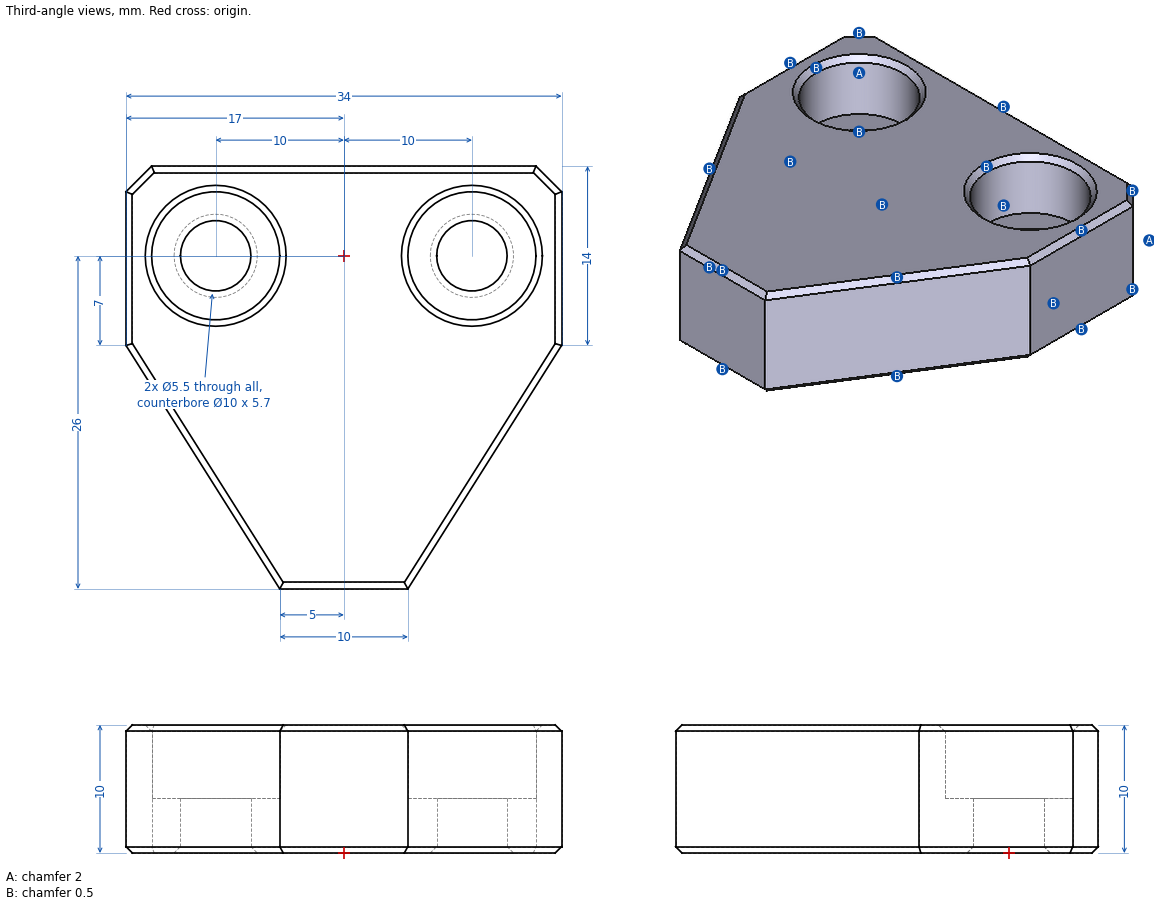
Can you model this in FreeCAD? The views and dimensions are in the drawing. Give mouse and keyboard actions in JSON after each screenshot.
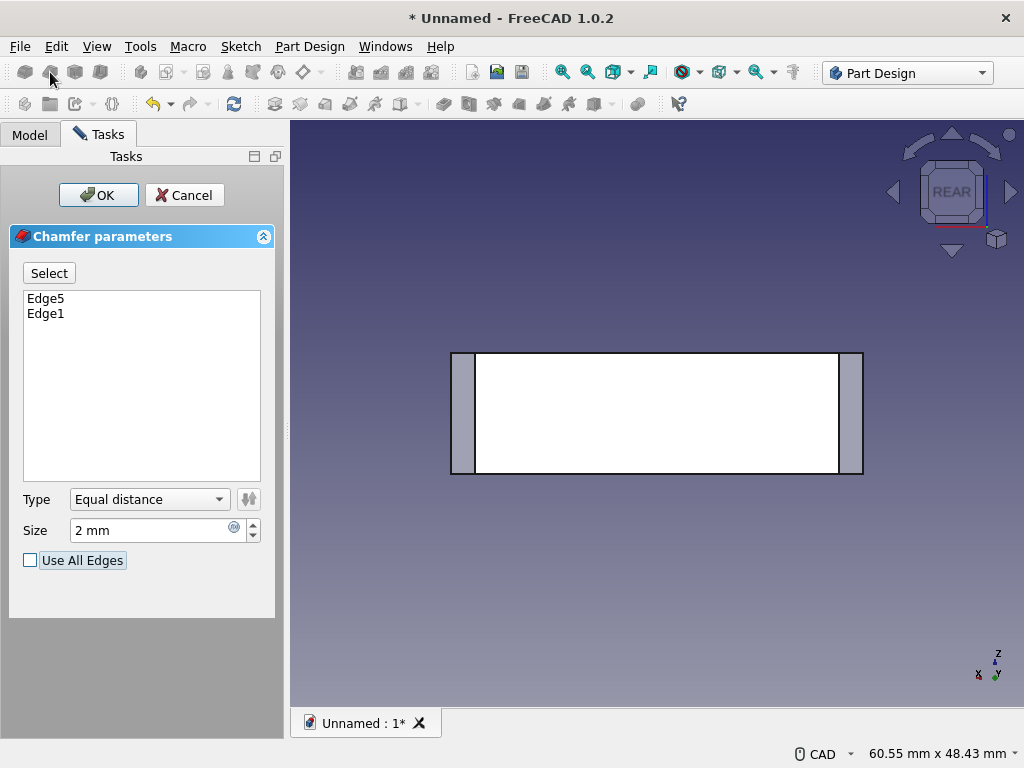
{"action": "left_click", "coordinate": [99, 195]}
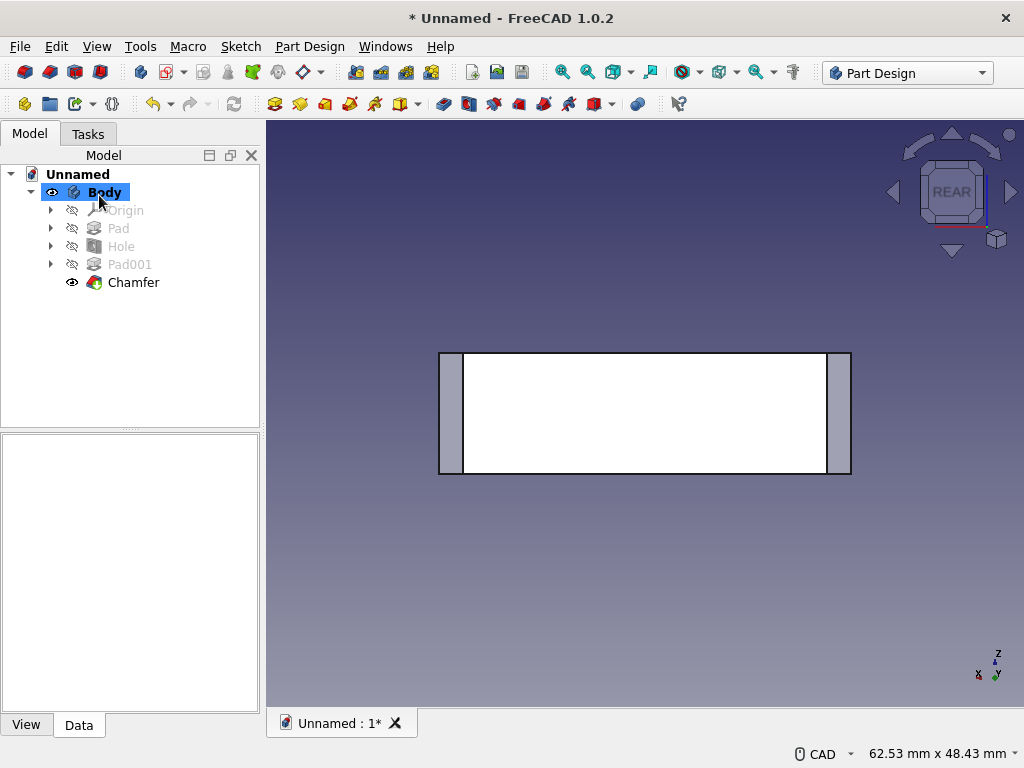
{"action": "key", "text": "0"}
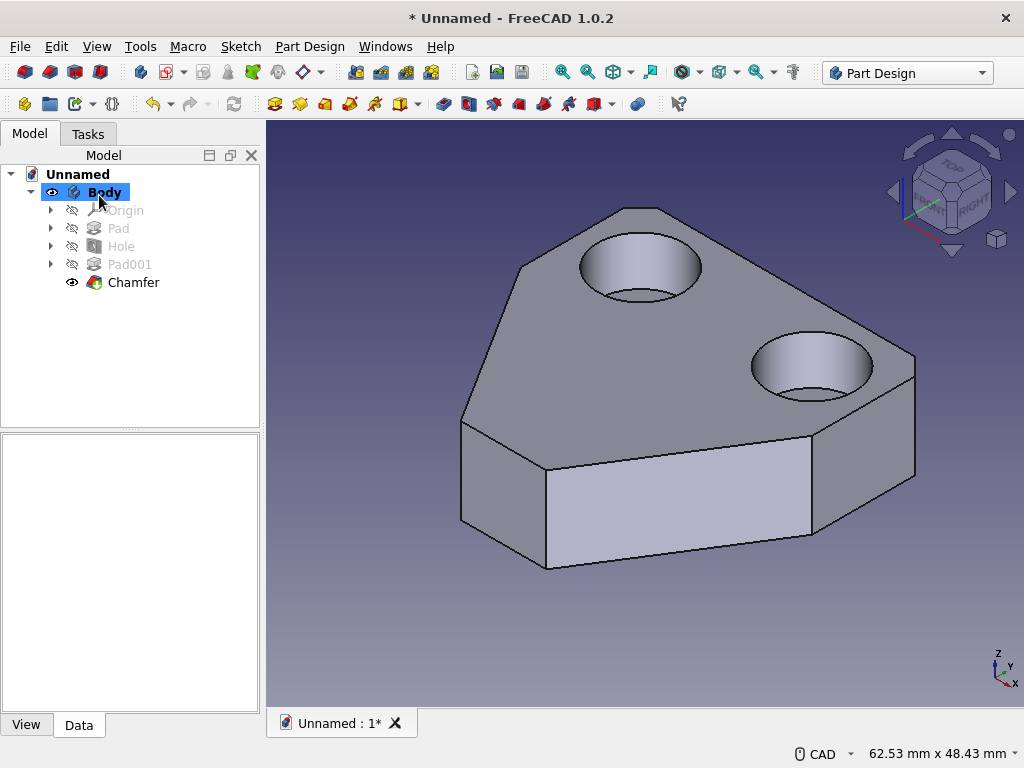
{"action": "left_click", "coordinate": [605, 386]}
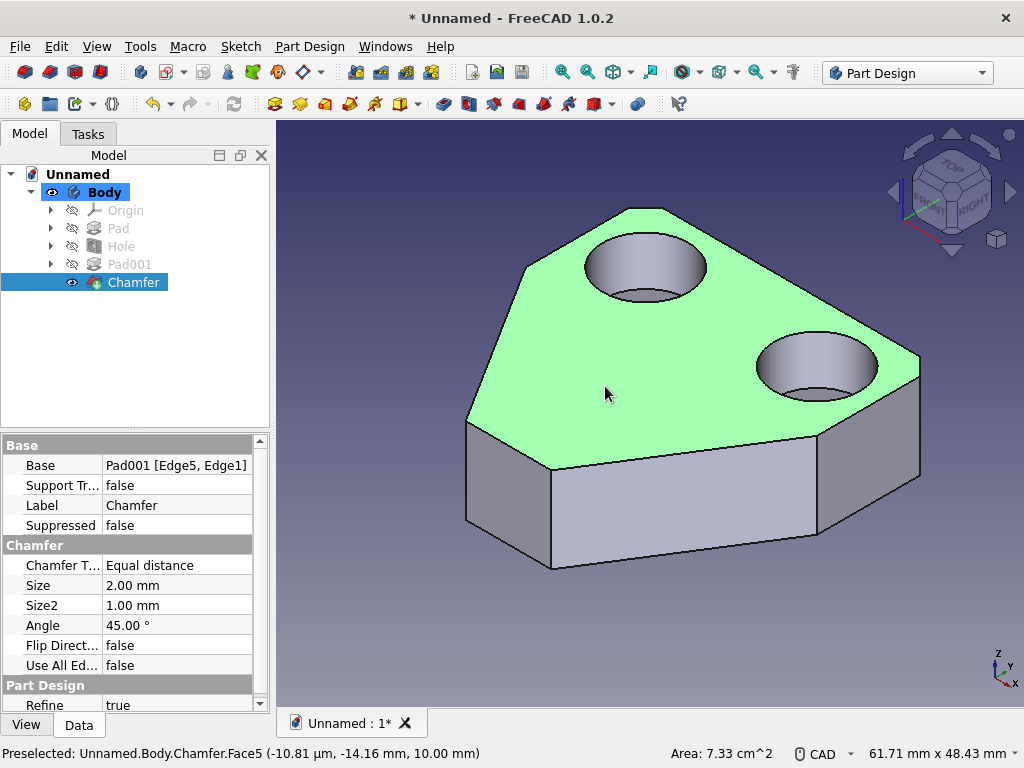
{"action": "key", "text": "2"}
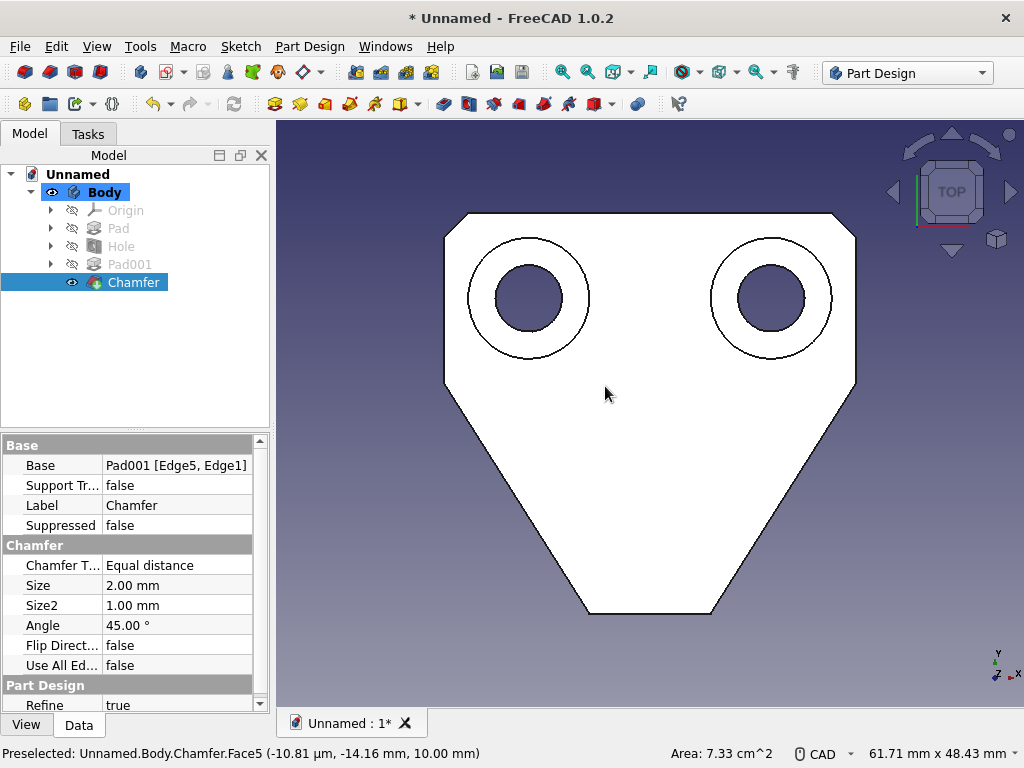
{"action": "key", "text": "1"}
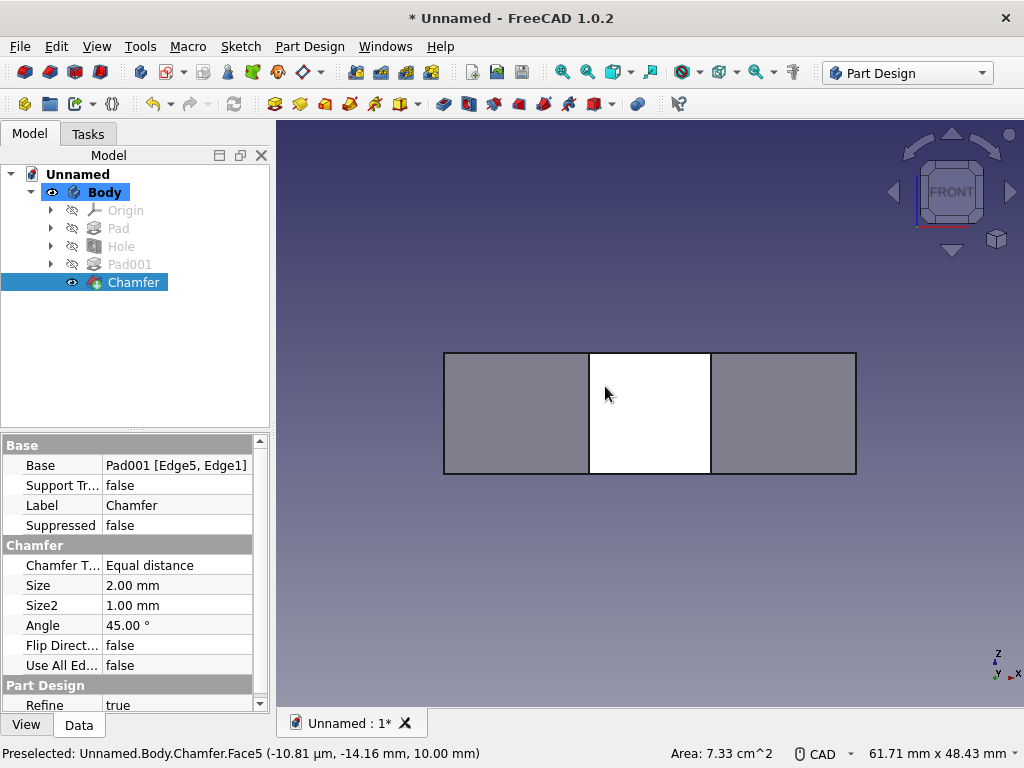
{"action": "key", "text": "3"}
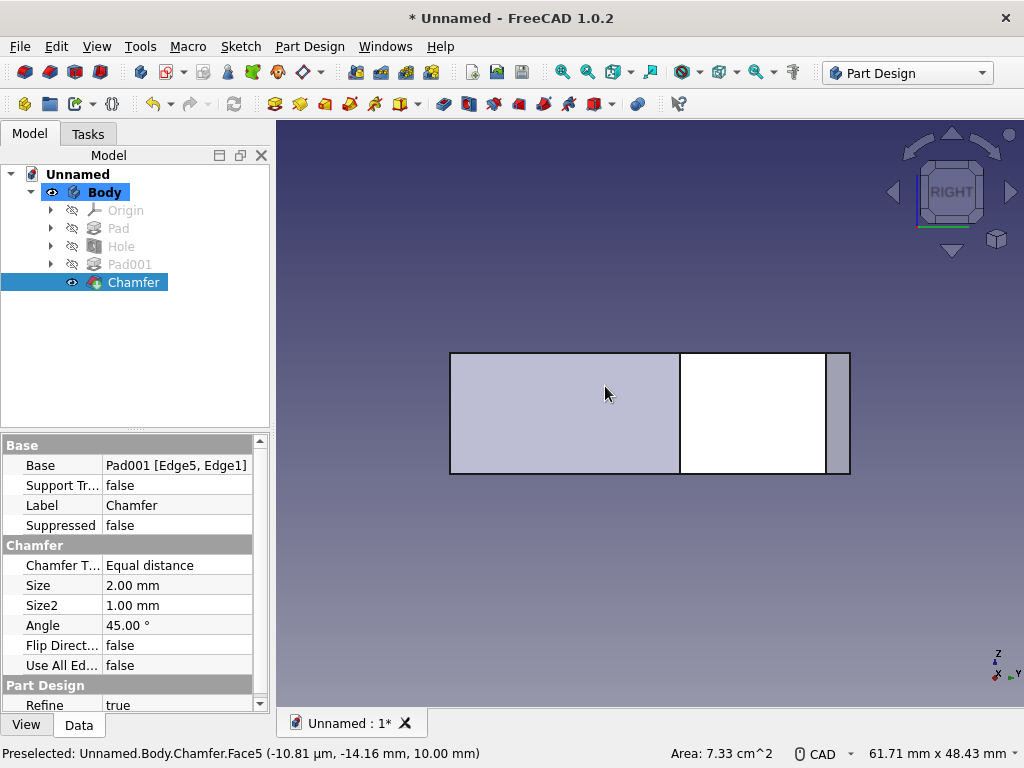
{"action": "key", "text": "5"}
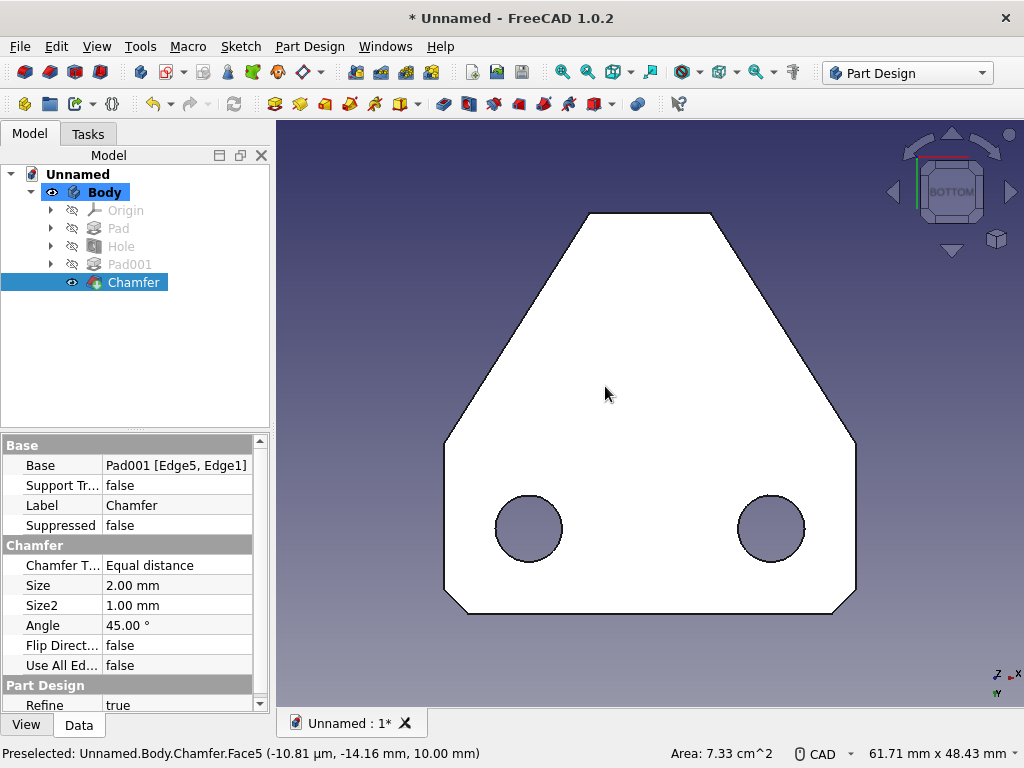
{"action": "left_click", "coordinate": [650, 412], "text": "ctrl"}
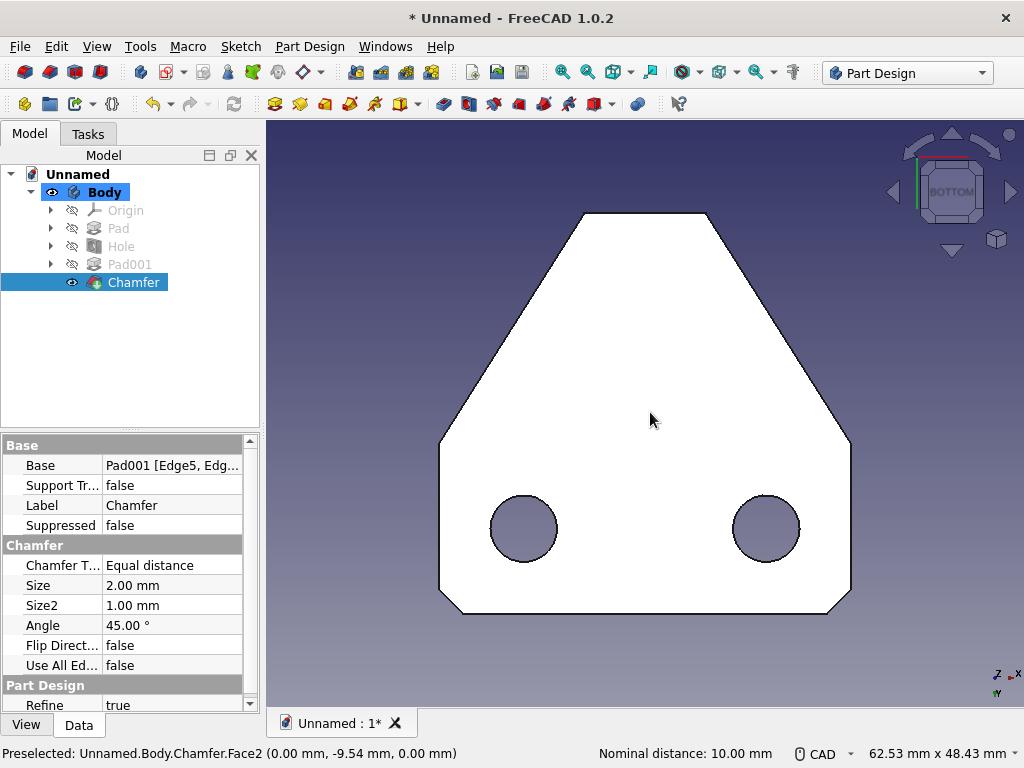
{"action": "left_click", "coordinate": [50, 72]}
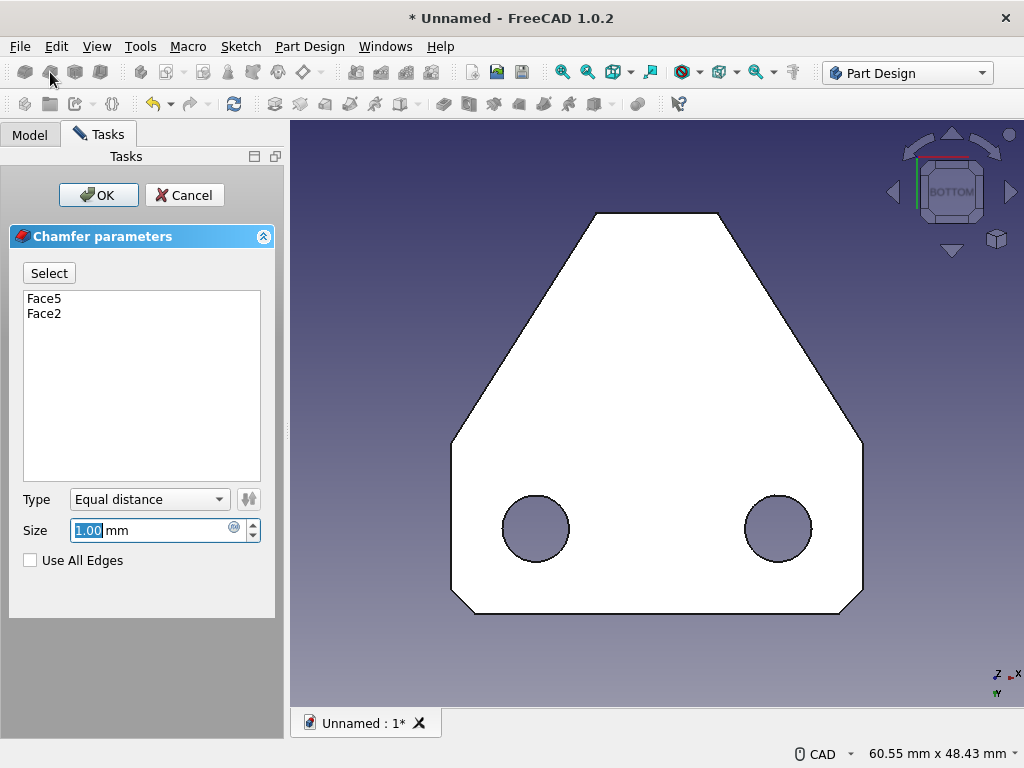
{"action": "type", "text": "0.5"}
{"action": "key", "text": "Tab"}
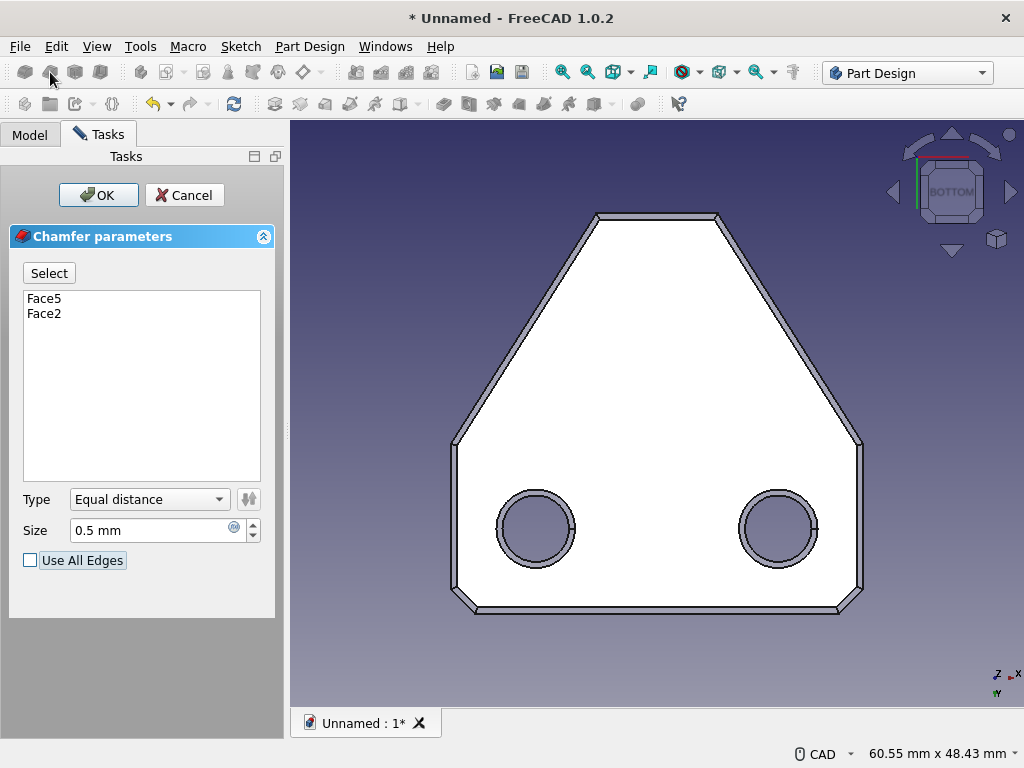
{"action": "left_click", "coordinate": [99, 195]}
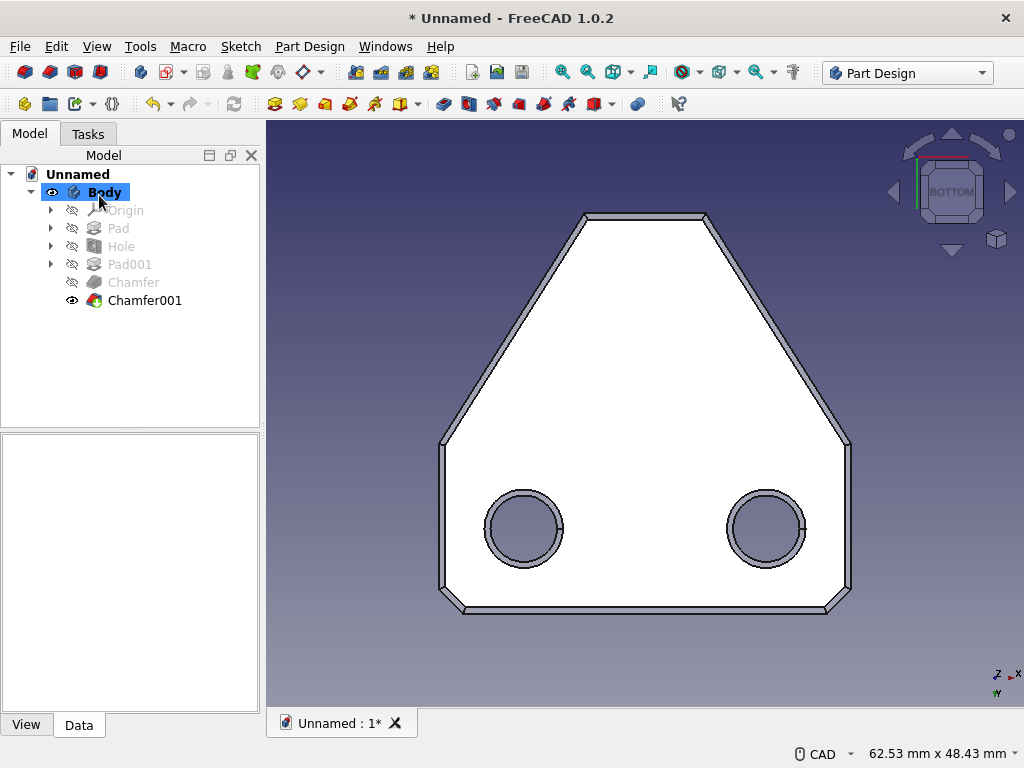
{"action": "key", "text": "0"}